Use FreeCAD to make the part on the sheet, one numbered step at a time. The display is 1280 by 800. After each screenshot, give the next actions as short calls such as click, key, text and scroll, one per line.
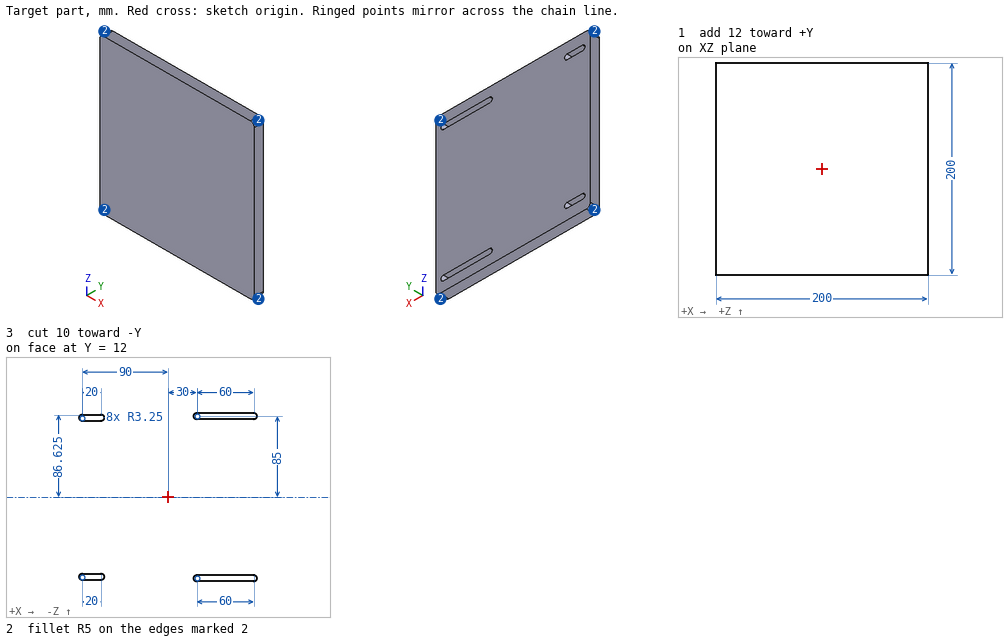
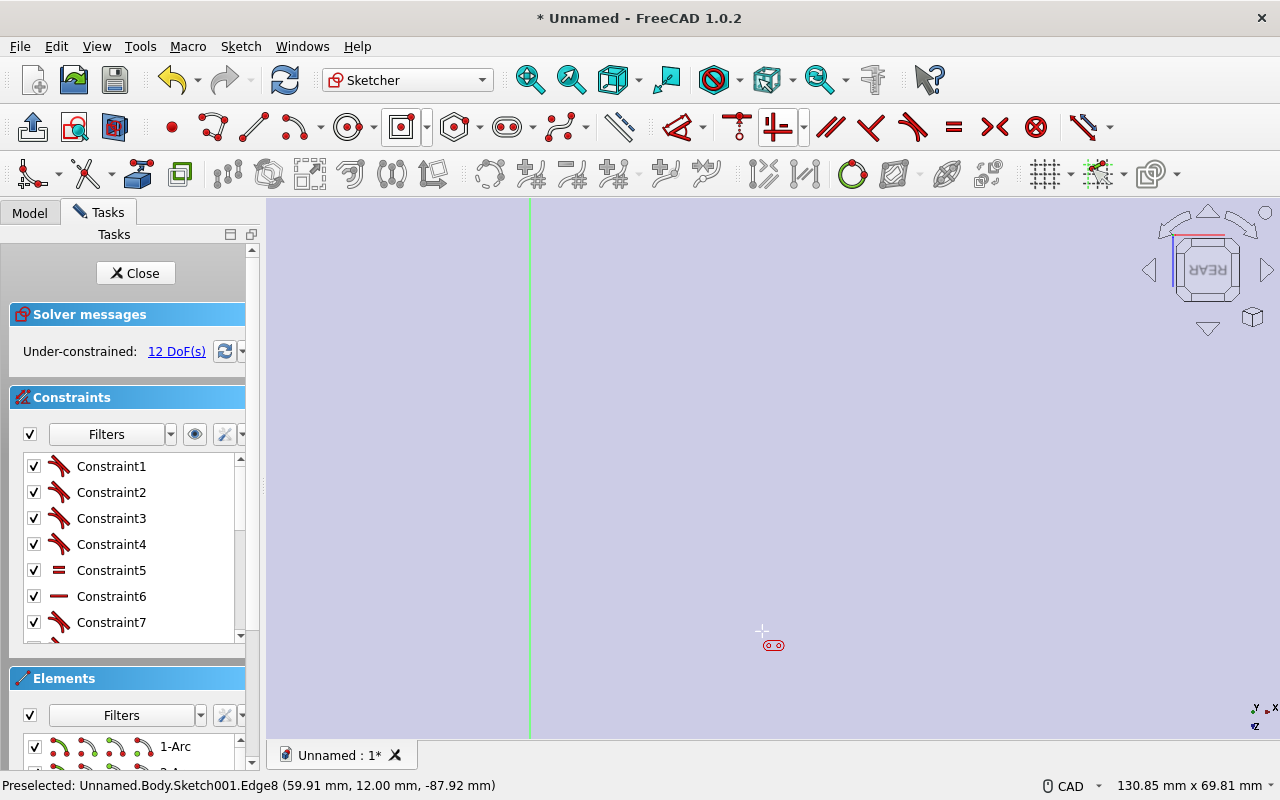
scroll(762, 632, down, 7)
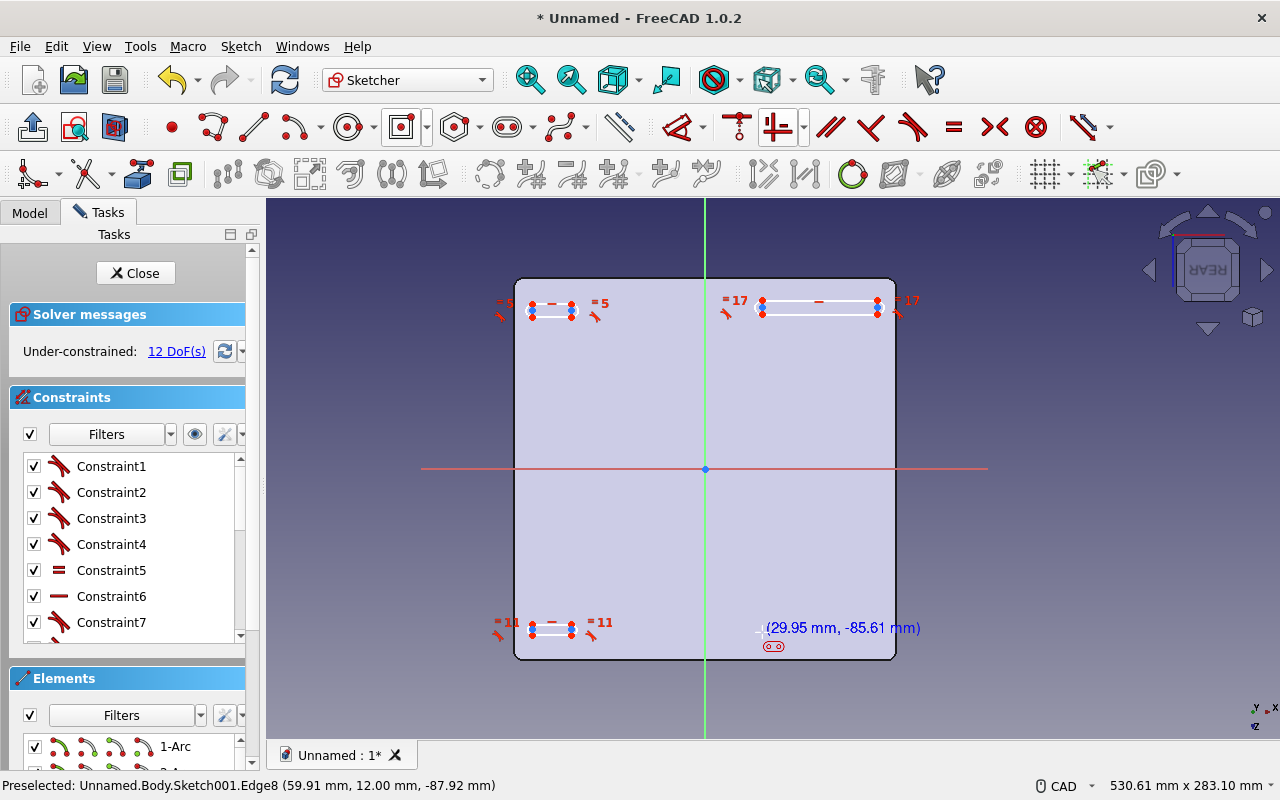
click(762, 632)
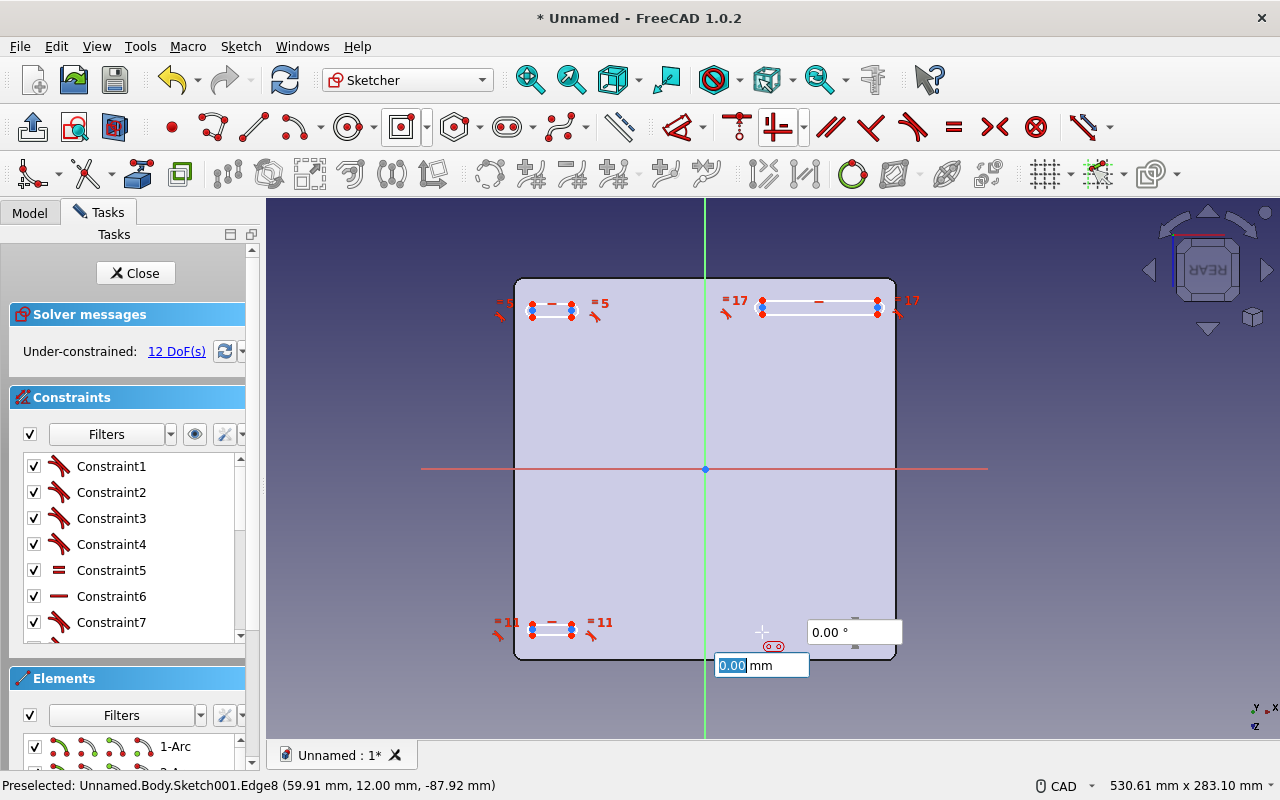
click(877, 632)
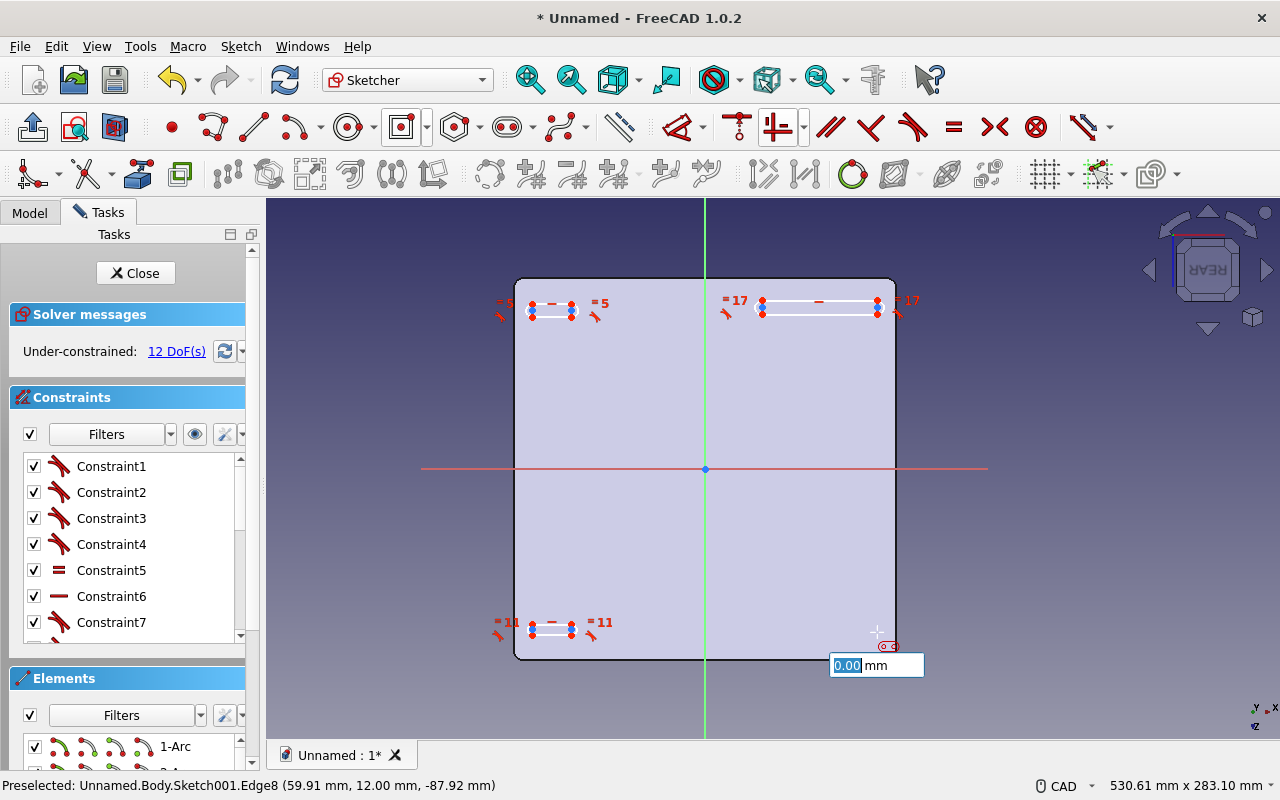
scroll(820, 638, up, 5)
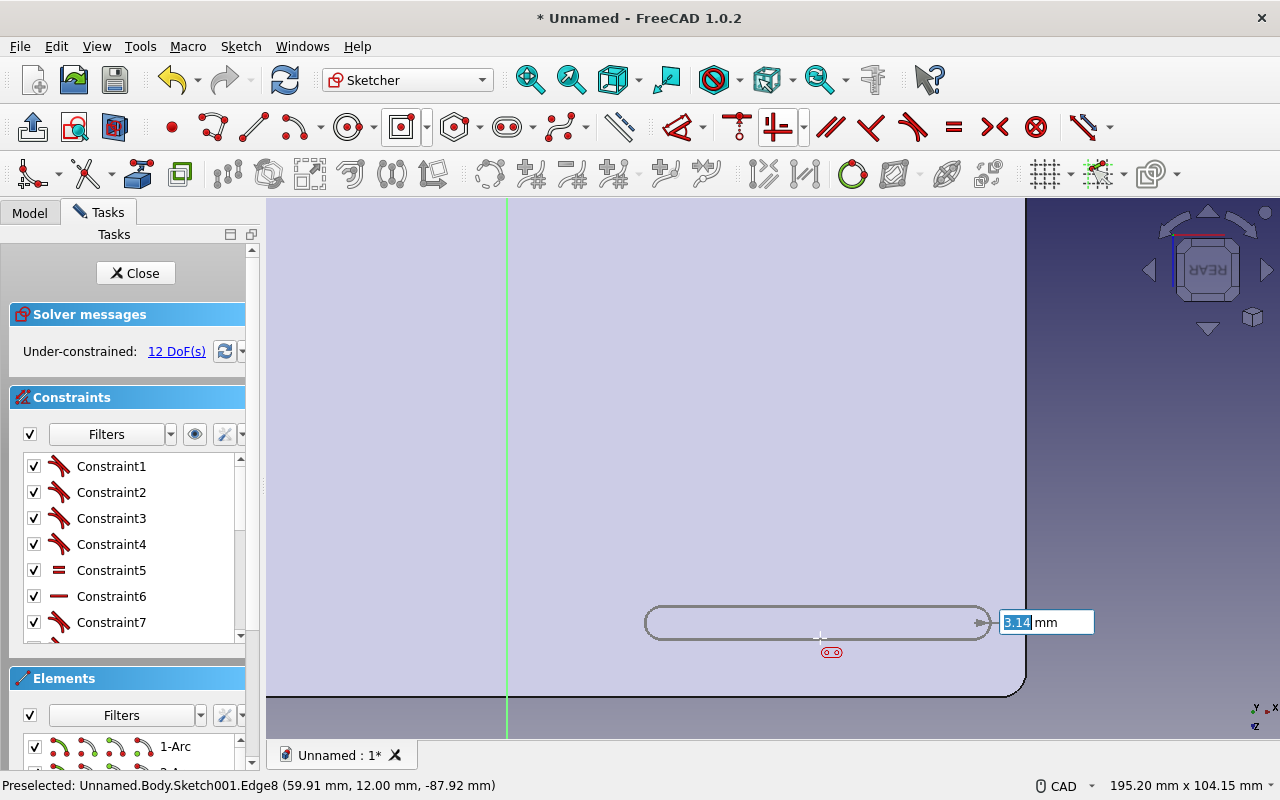
click(818, 636)
key(Escape)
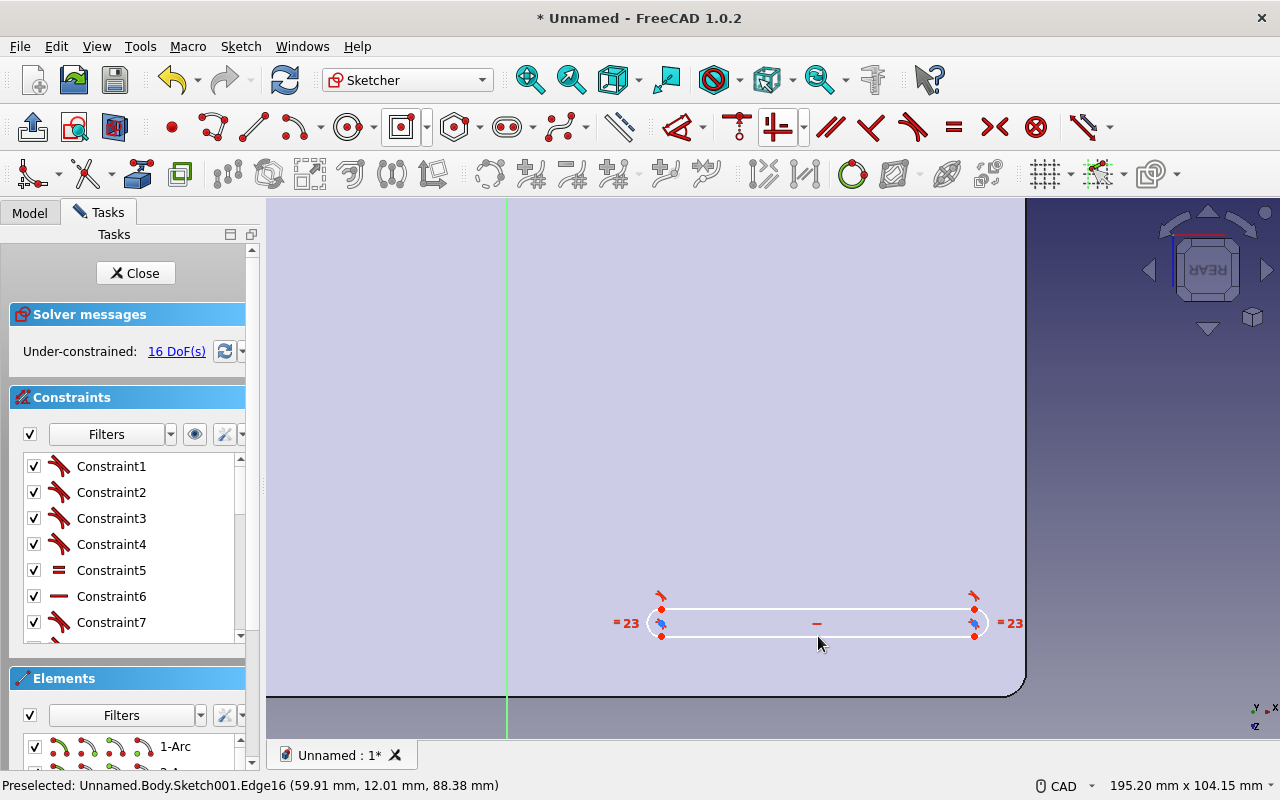
scroll(820, 638, down, 5)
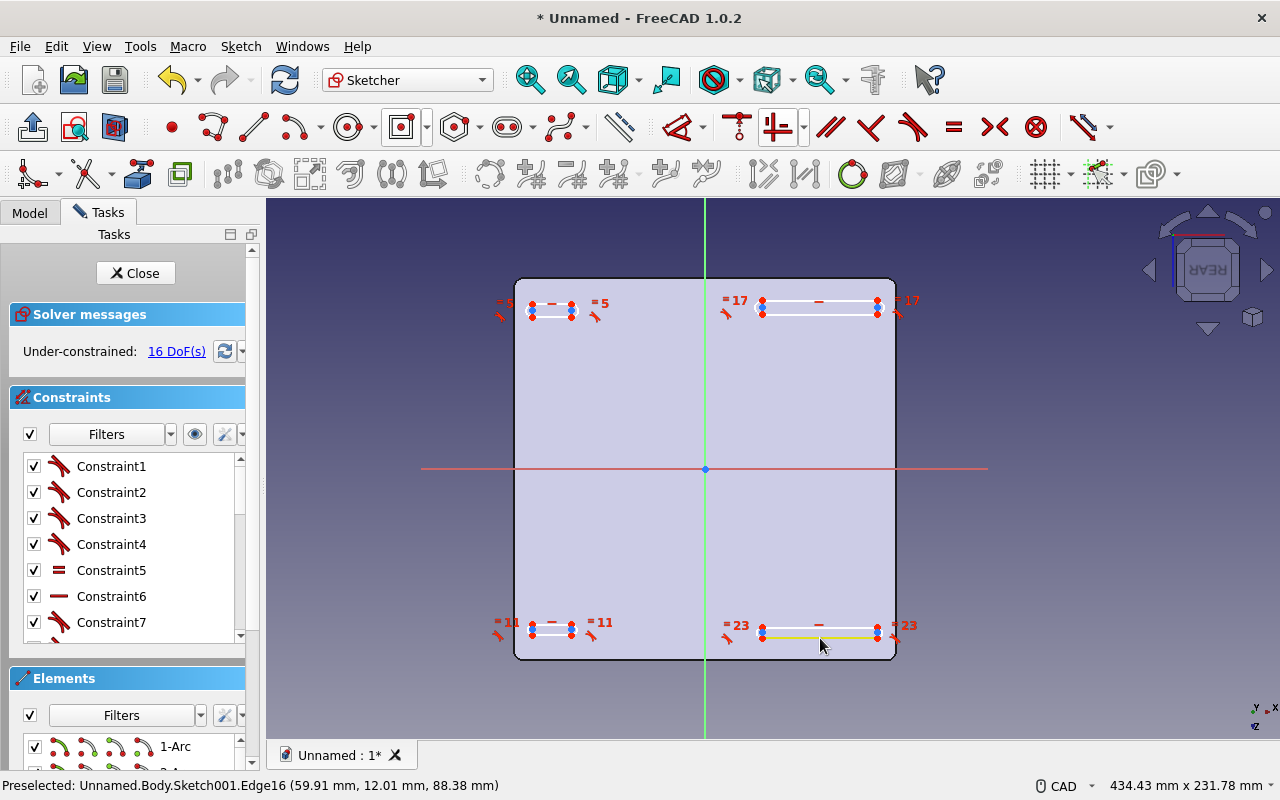
scroll(527, 307, up, 5)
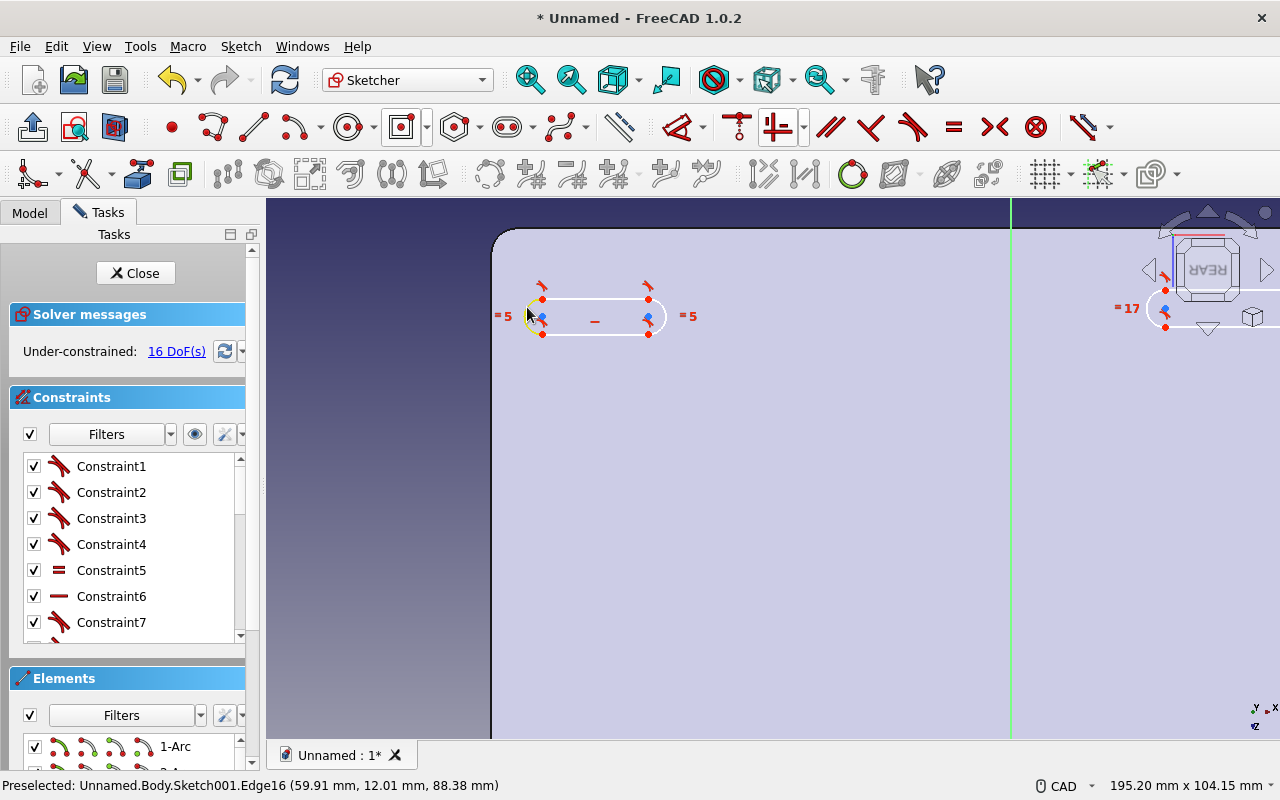
click(528, 306)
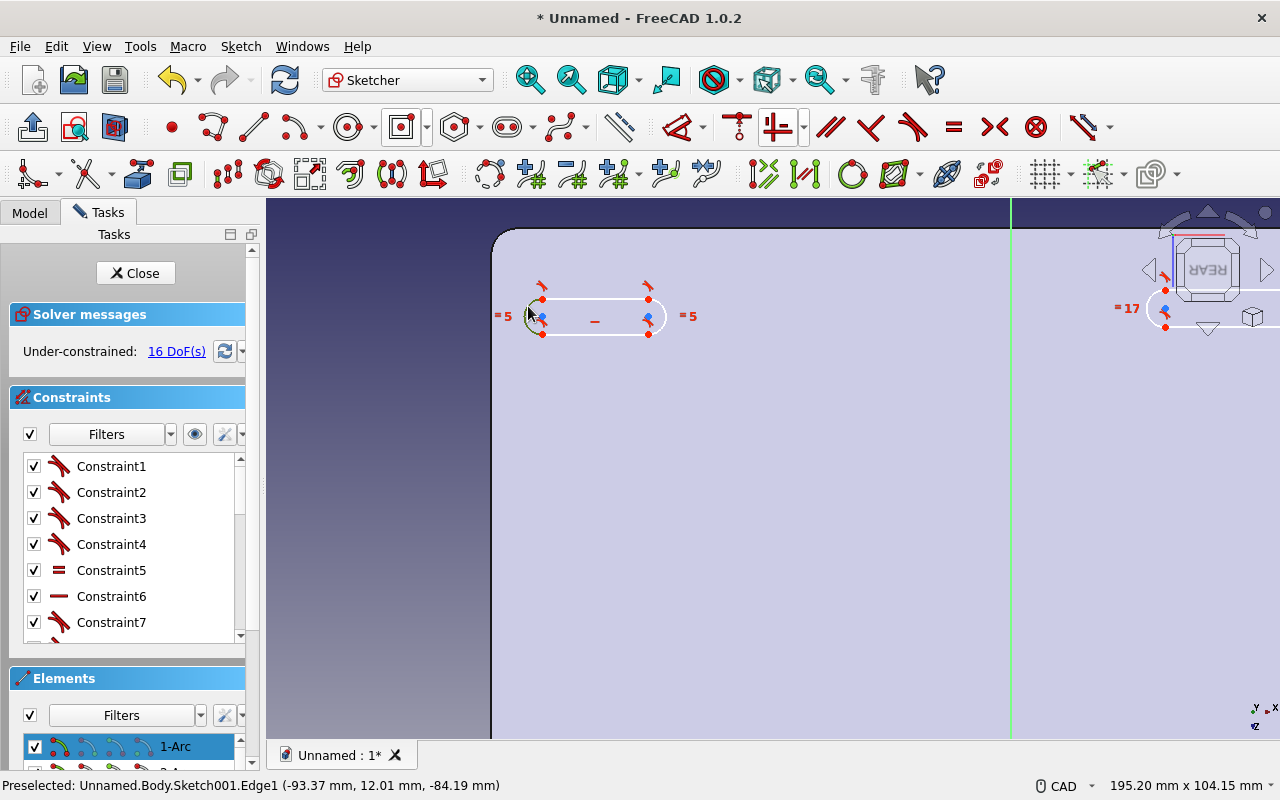
scroll(526, 306, down, 5)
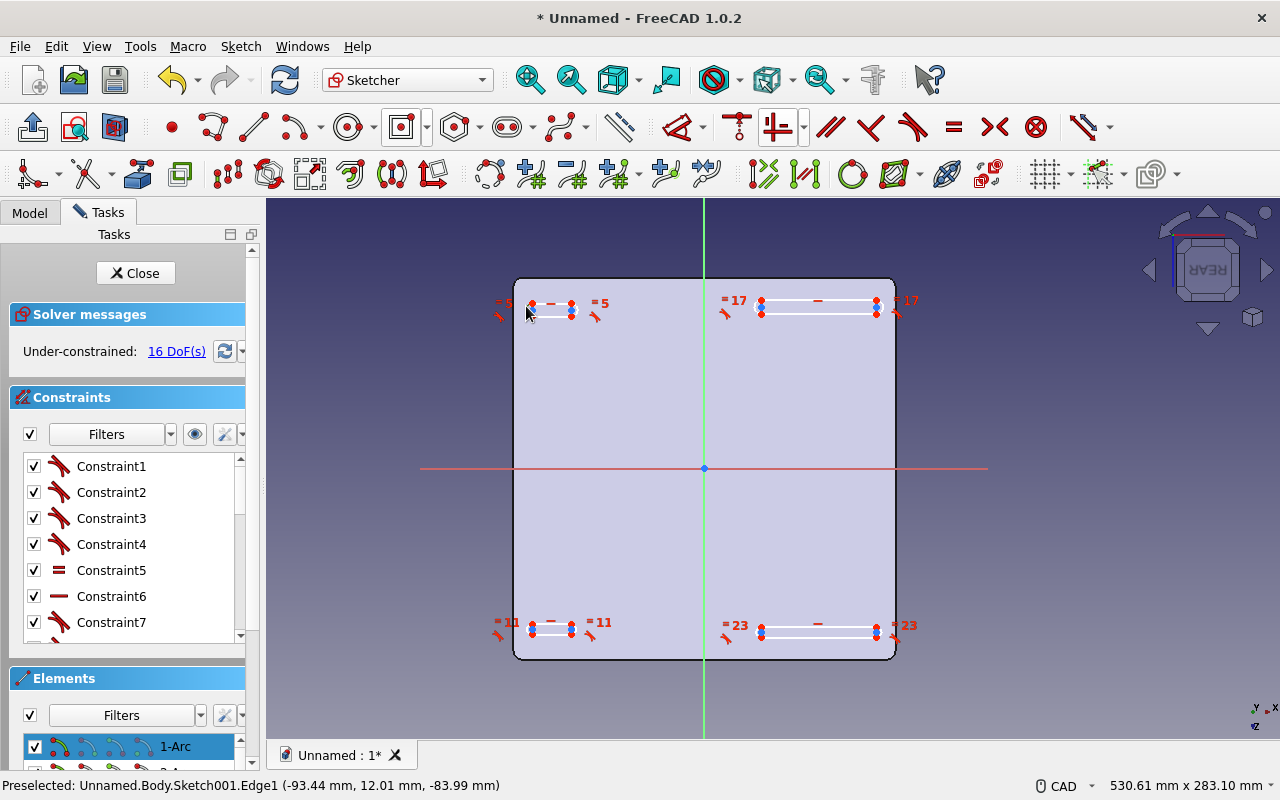
scroll(528, 626, up, 6)